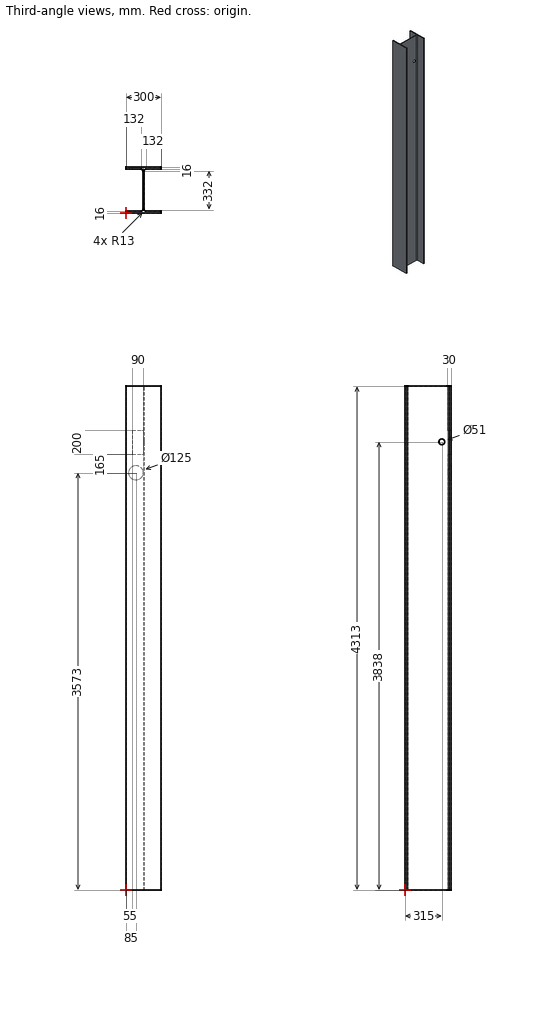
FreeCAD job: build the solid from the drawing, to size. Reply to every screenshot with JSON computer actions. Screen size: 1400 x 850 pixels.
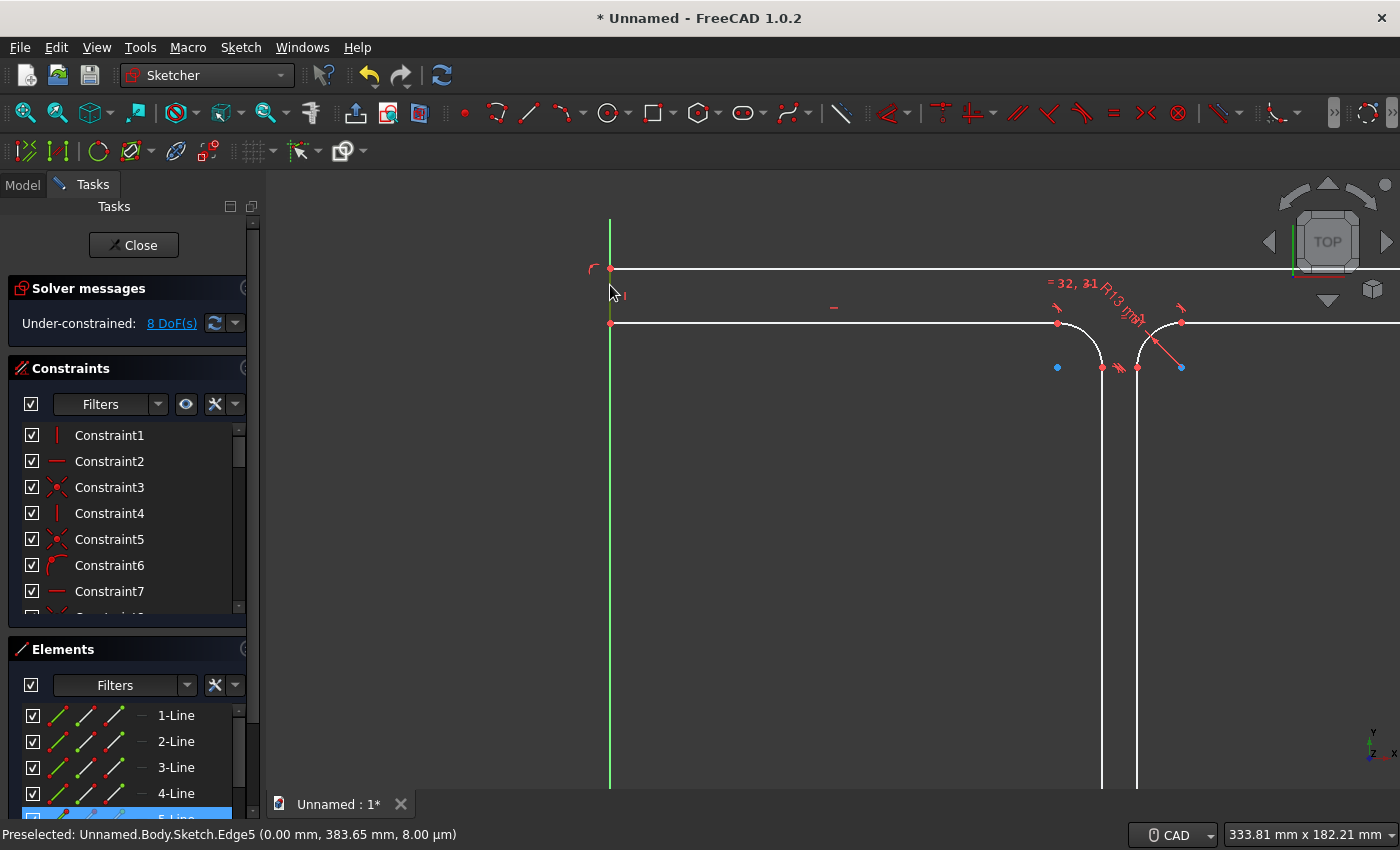
{"action": "key", "text": "i"}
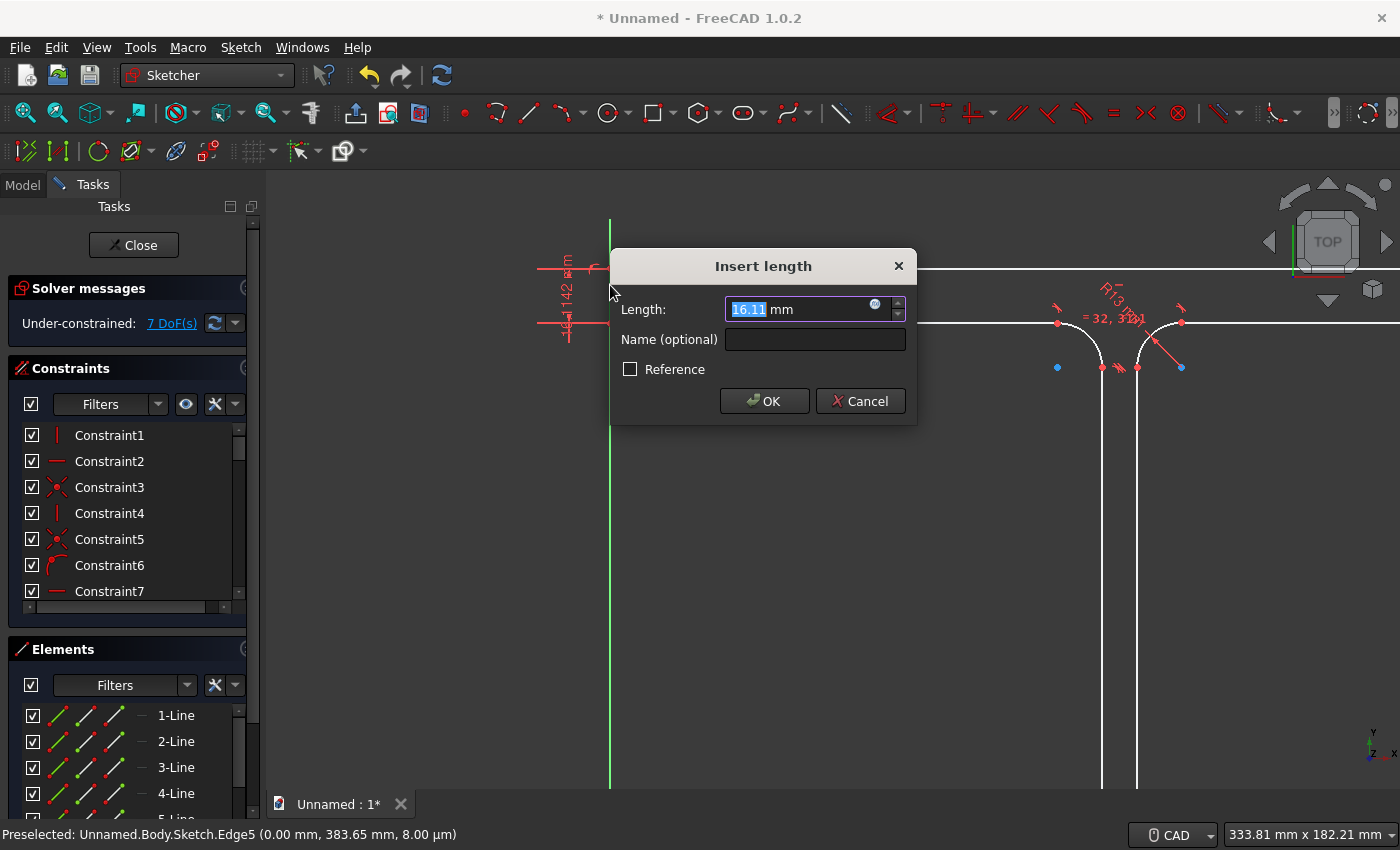
{"action": "type", "text": "16"}
{"action": "key", "text": "Return"}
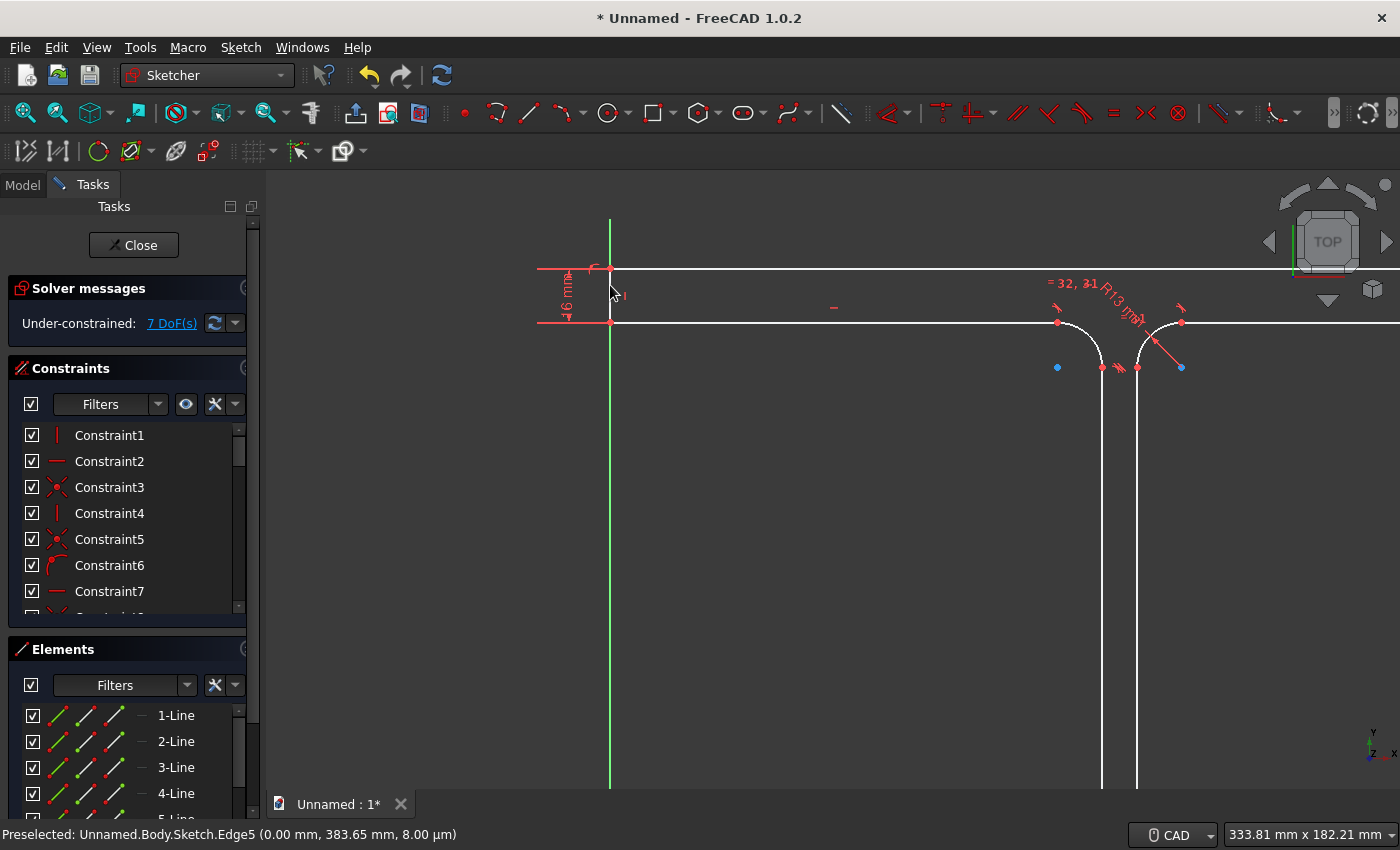
{"action": "scroll", "coordinate": [611, 287], "scroll_direction": "down", "scroll_amount": 6}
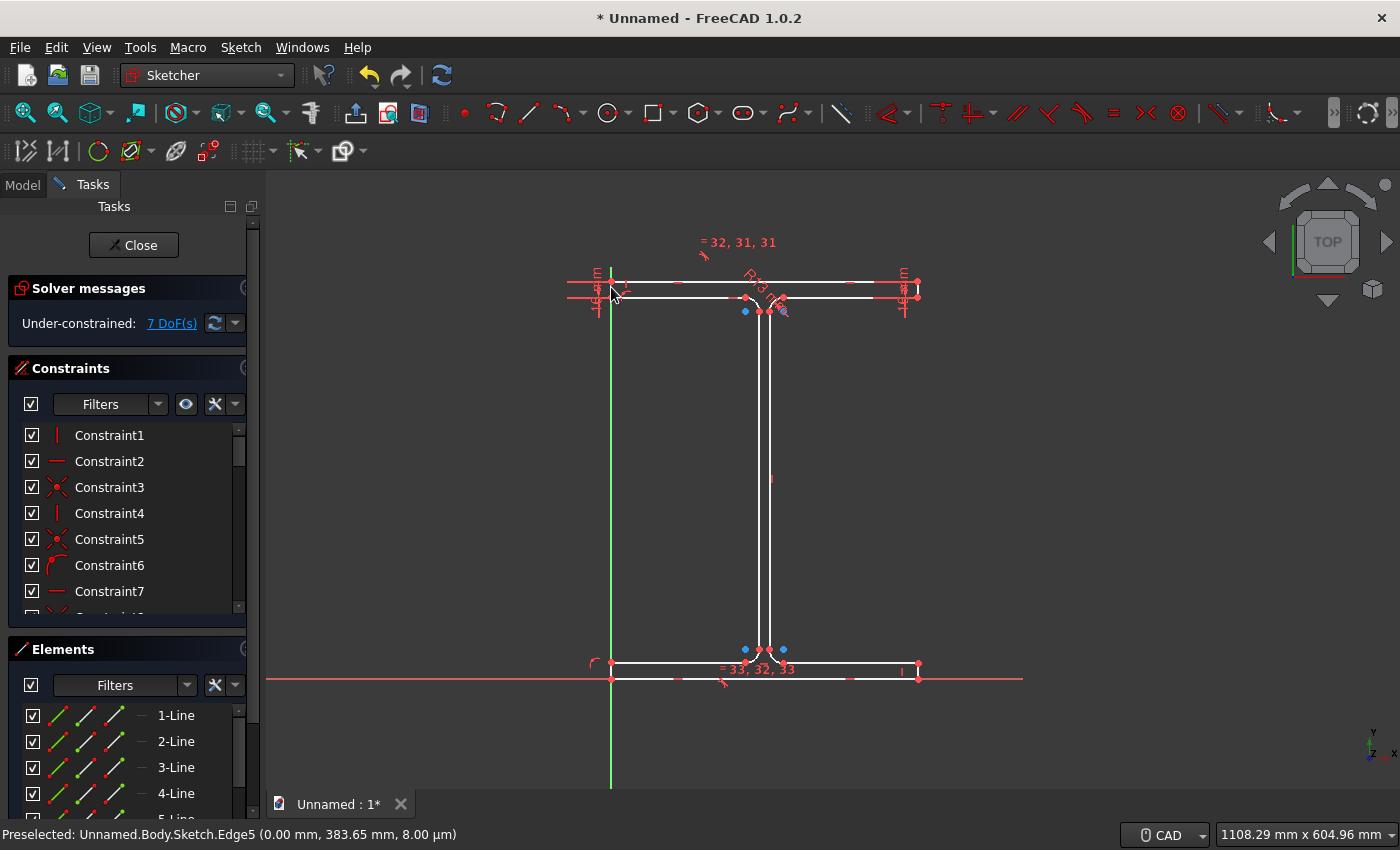
{"action": "scroll", "coordinate": [611, 668], "scroll_direction": "up", "scroll_amount": 6}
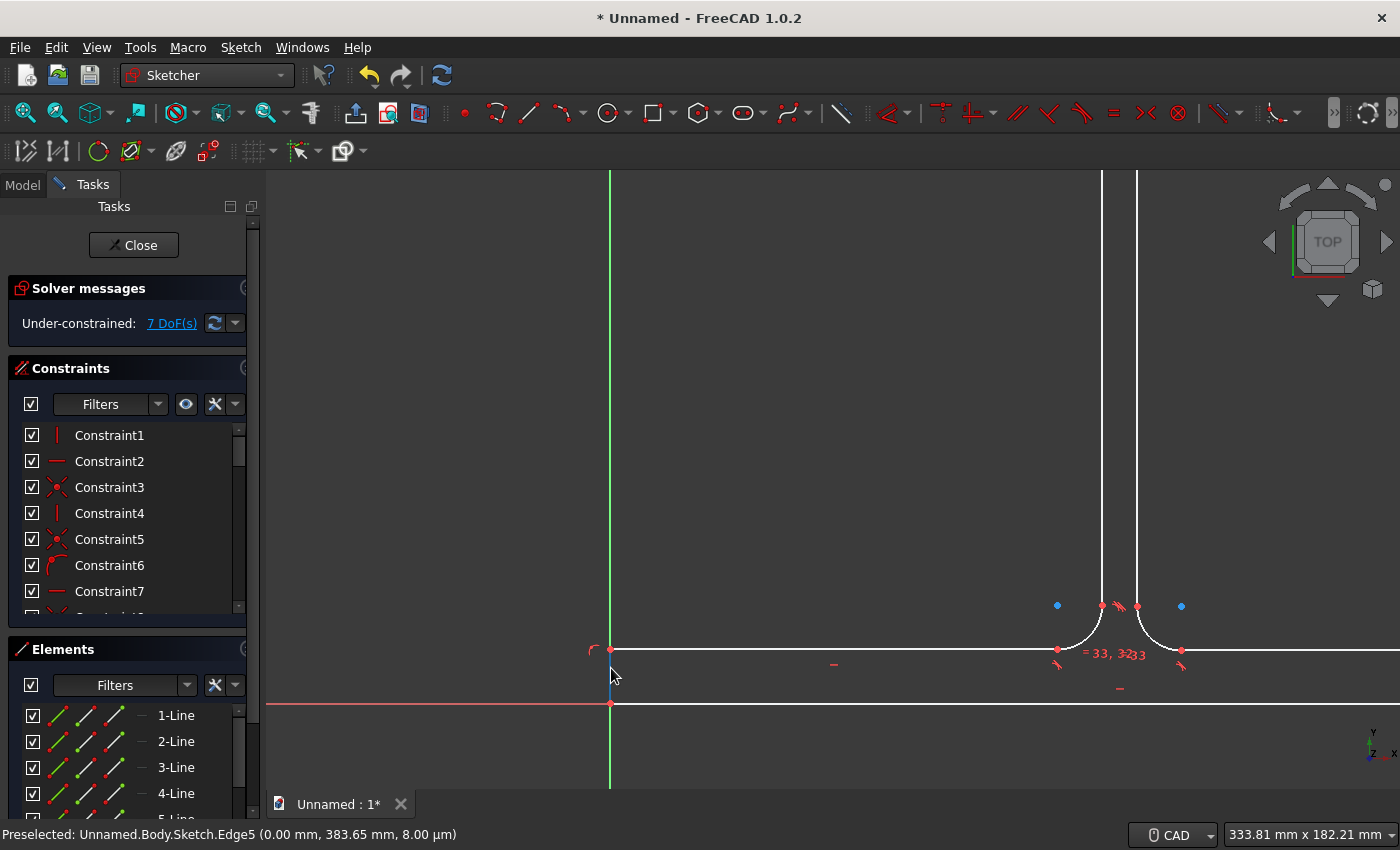
{"action": "left_click", "coordinate": [610, 666]}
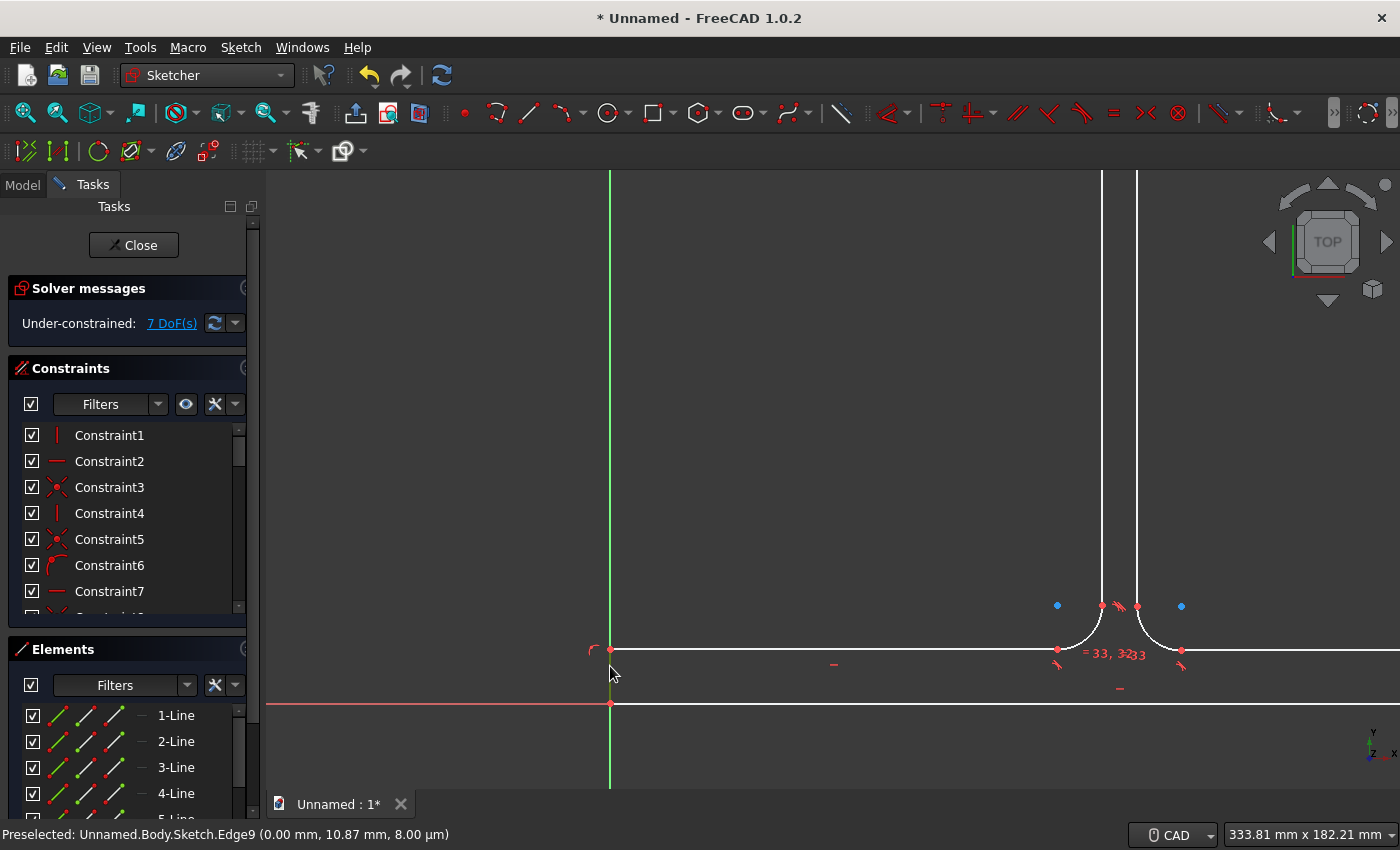
{"action": "left_click", "coordinate": [910, 114]}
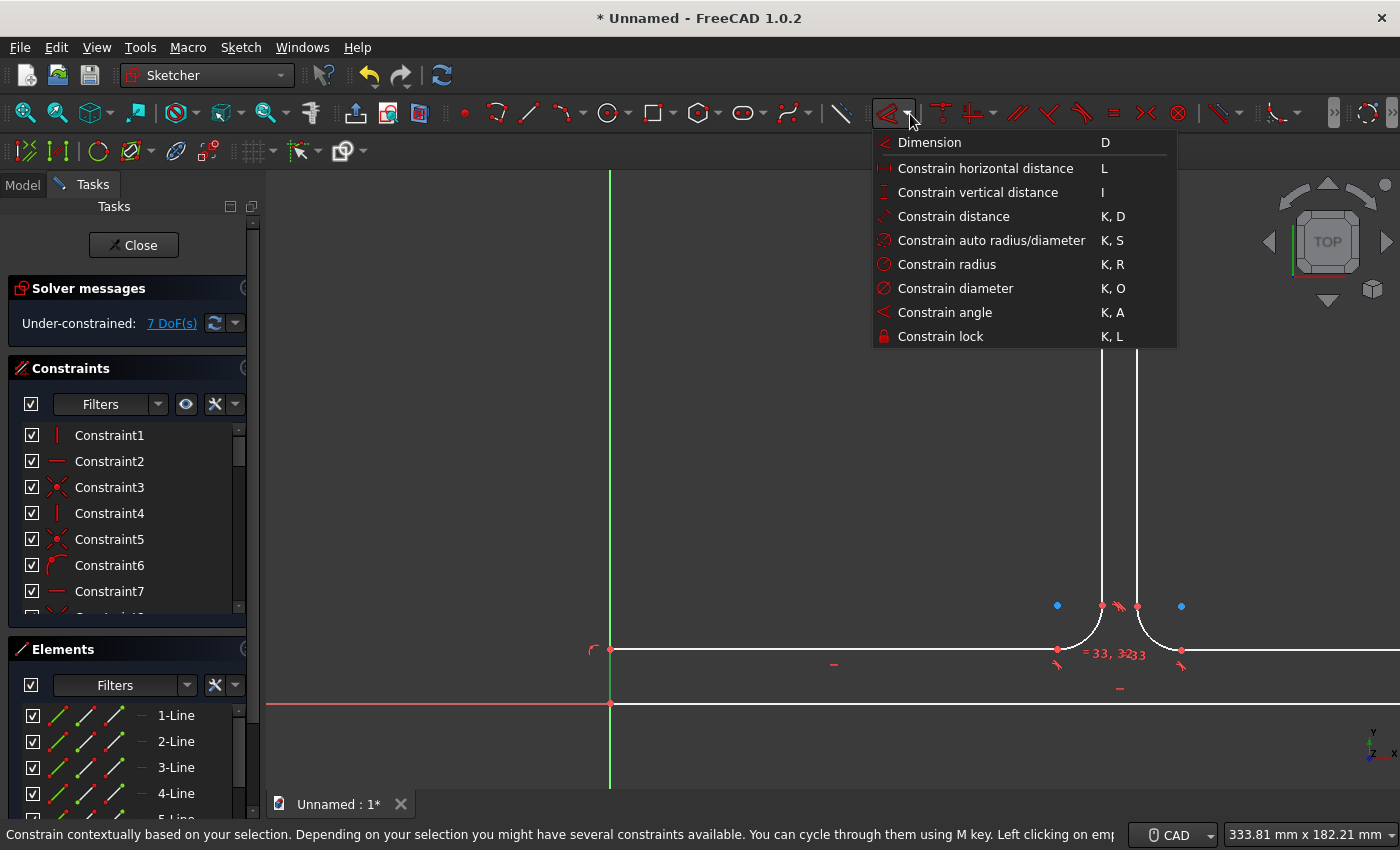
{"action": "left_click", "coordinate": [1025, 192]}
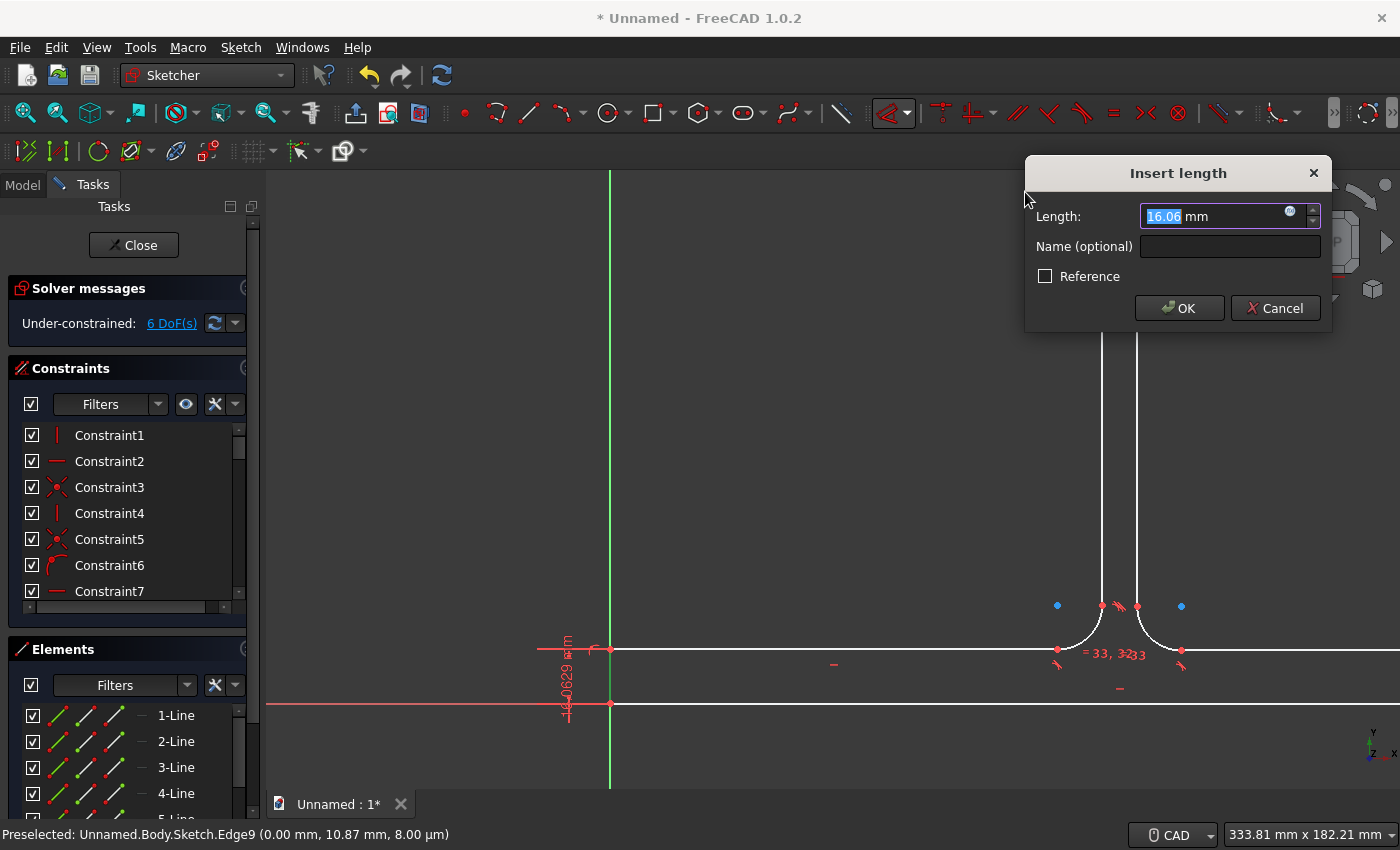
{"action": "type", "text": "16"}
{"action": "key", "text": "Return"}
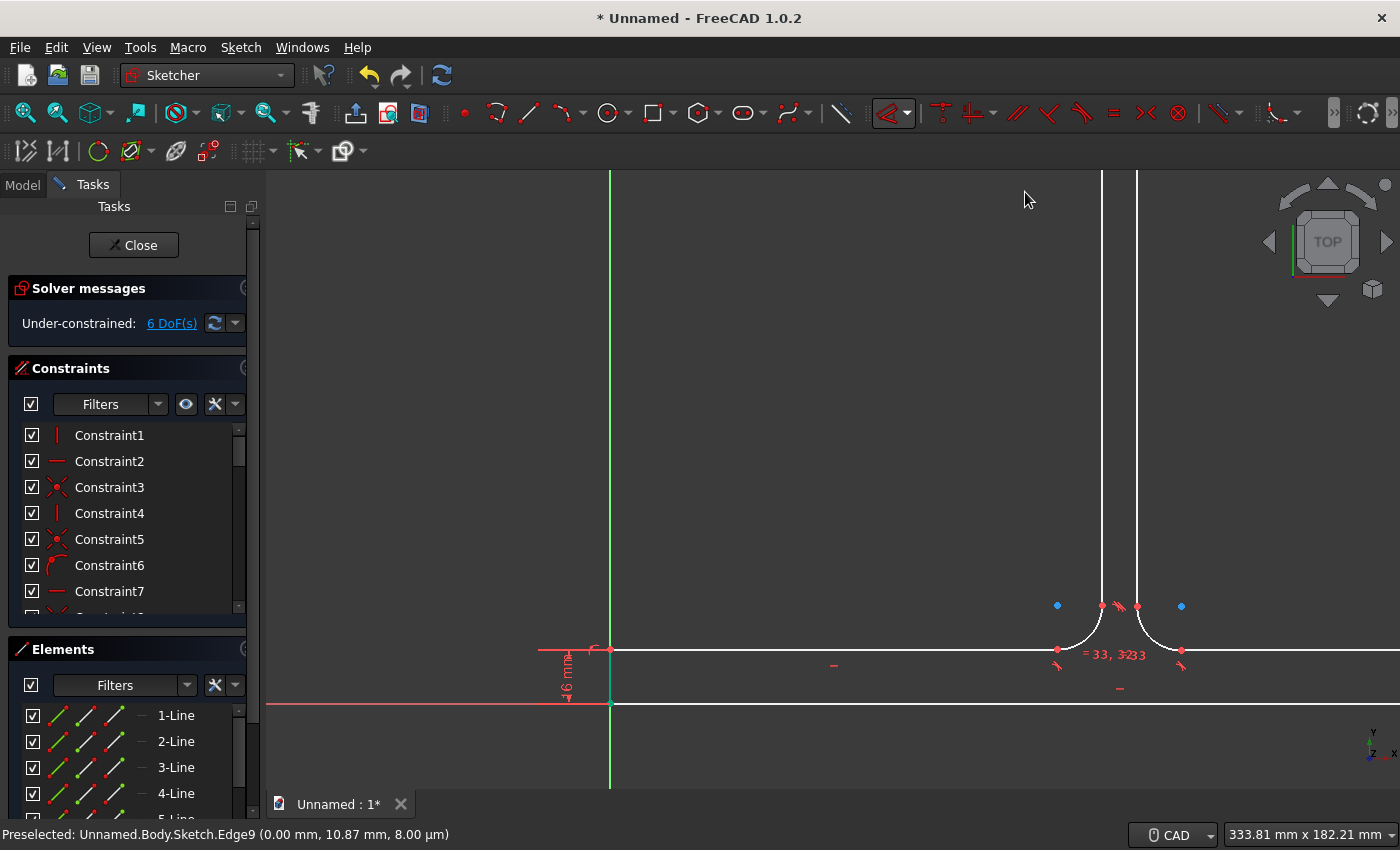
{"action": "scroll", "coordinate": [611, 668], "scroll_direction": "down", "scroll_amount": 6}